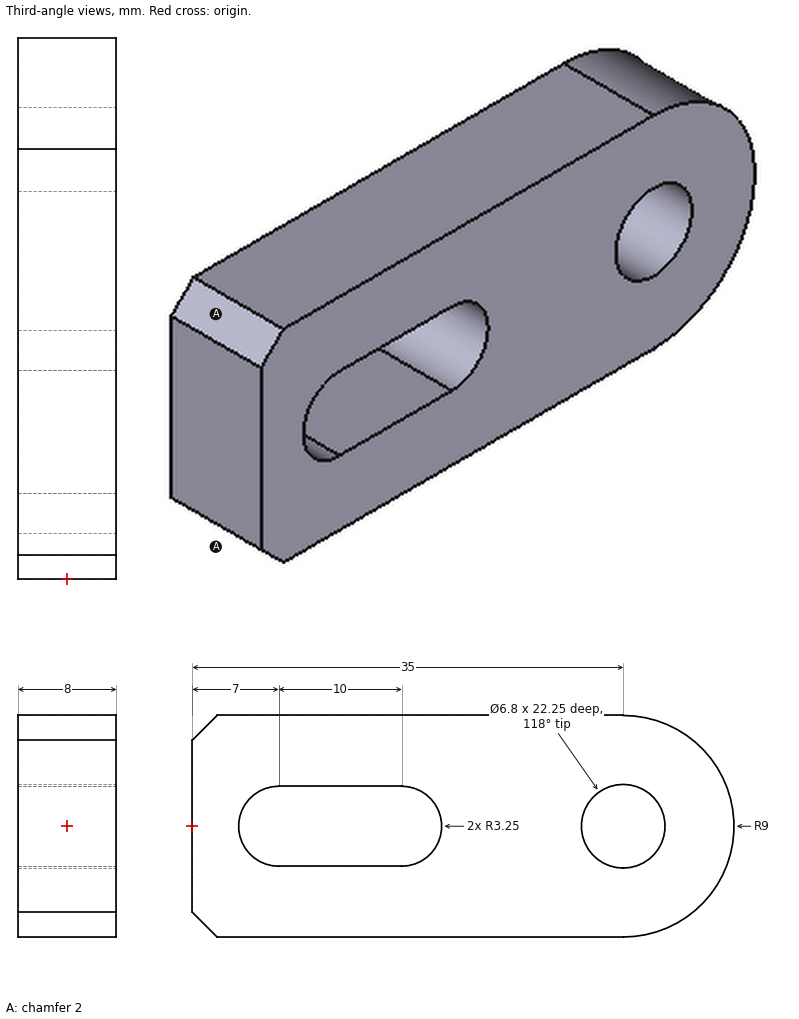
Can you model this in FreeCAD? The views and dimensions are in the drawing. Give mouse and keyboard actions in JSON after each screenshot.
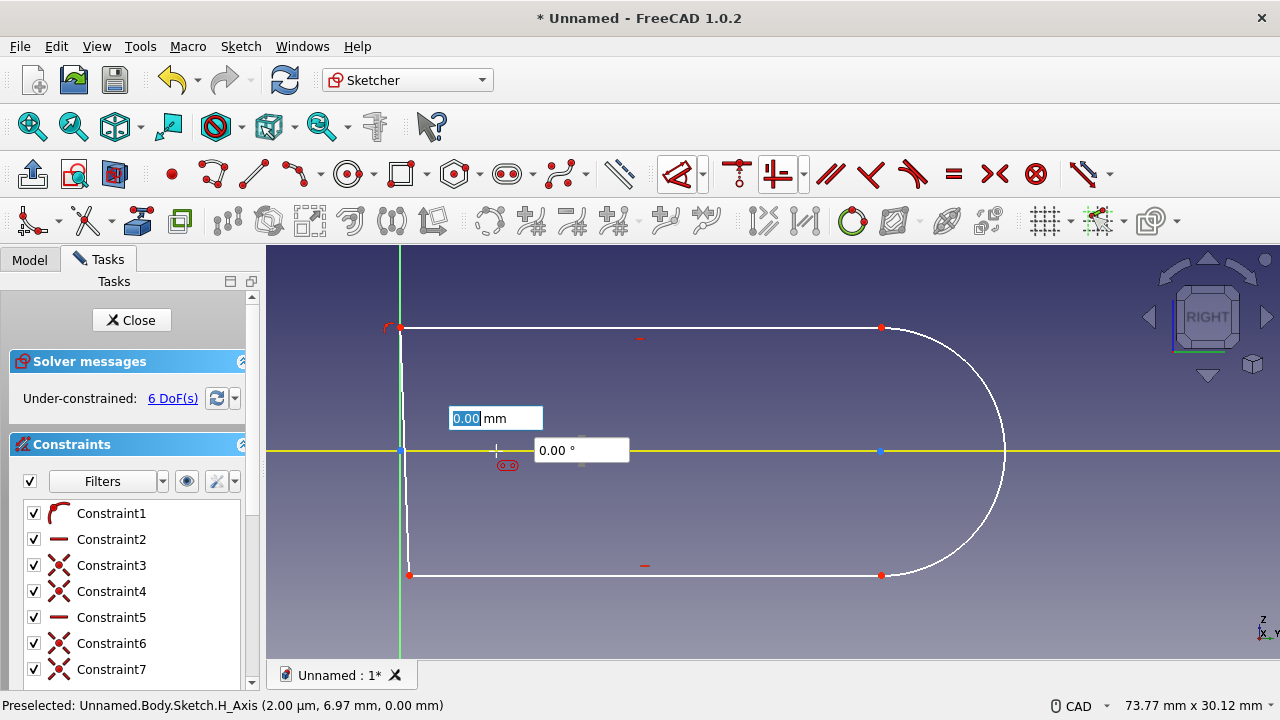
{"action": "left_click", "coordinate": [634, 442]}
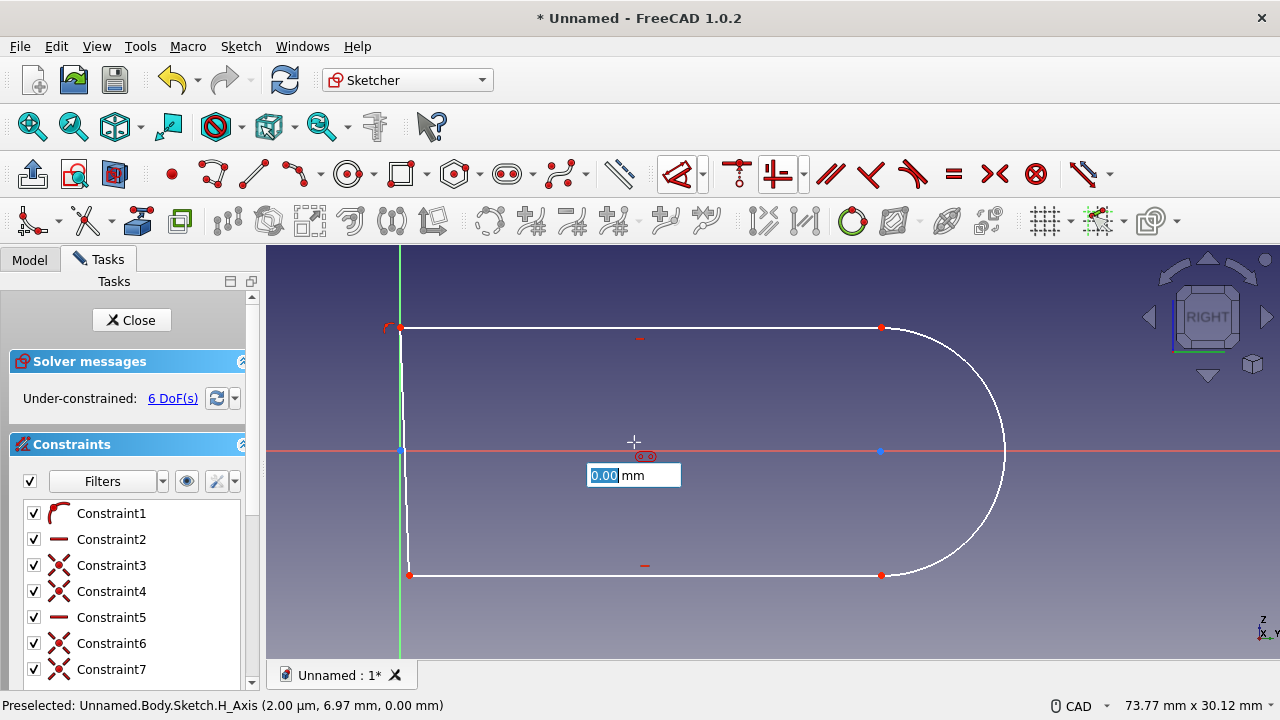
{"action": "left_click", "coordinate": [565, 496]}
{"action": "key", "text": "Escape"}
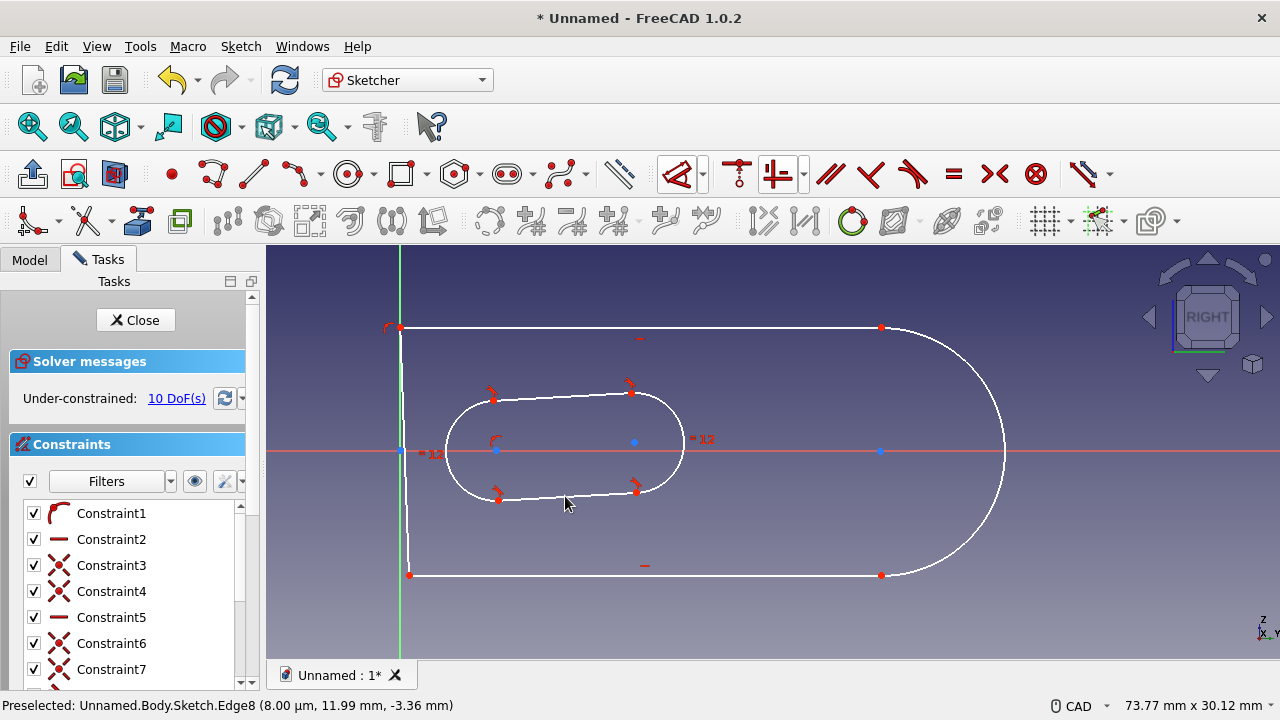
{"action": "left_click", "coordinate": [737, 328]}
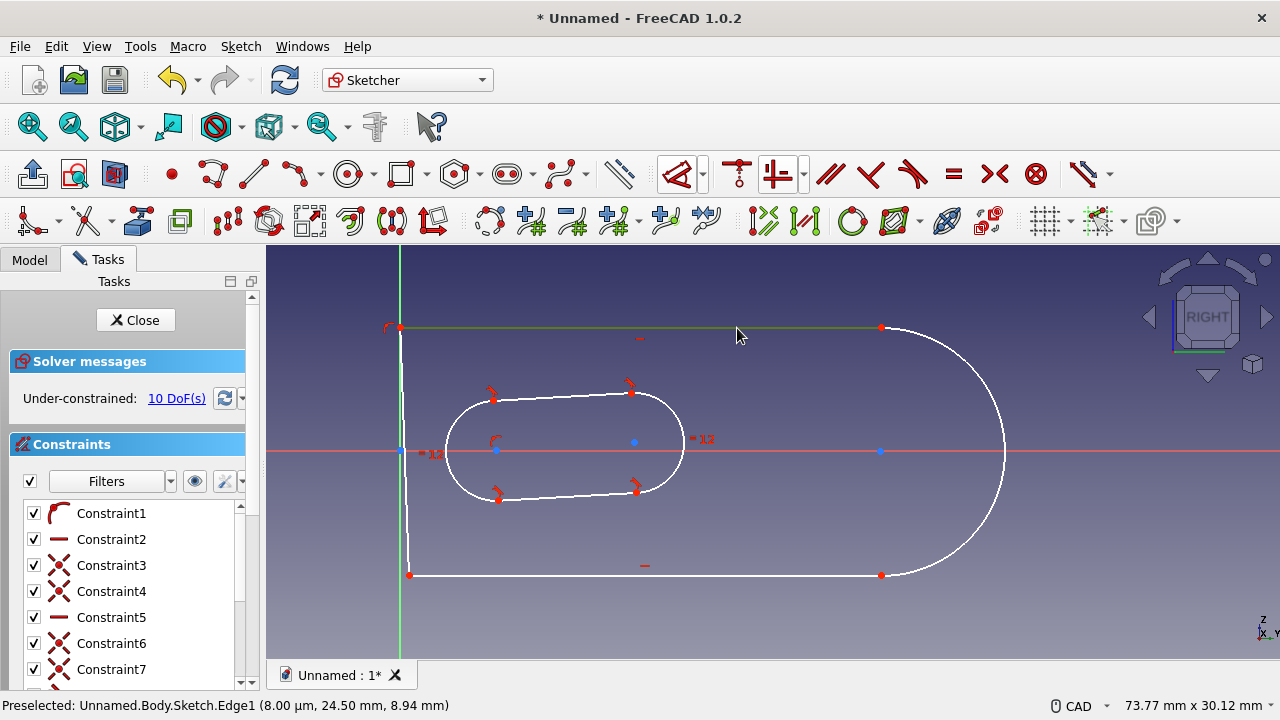
{"action": "left_click", "coordinate": [981, 525]}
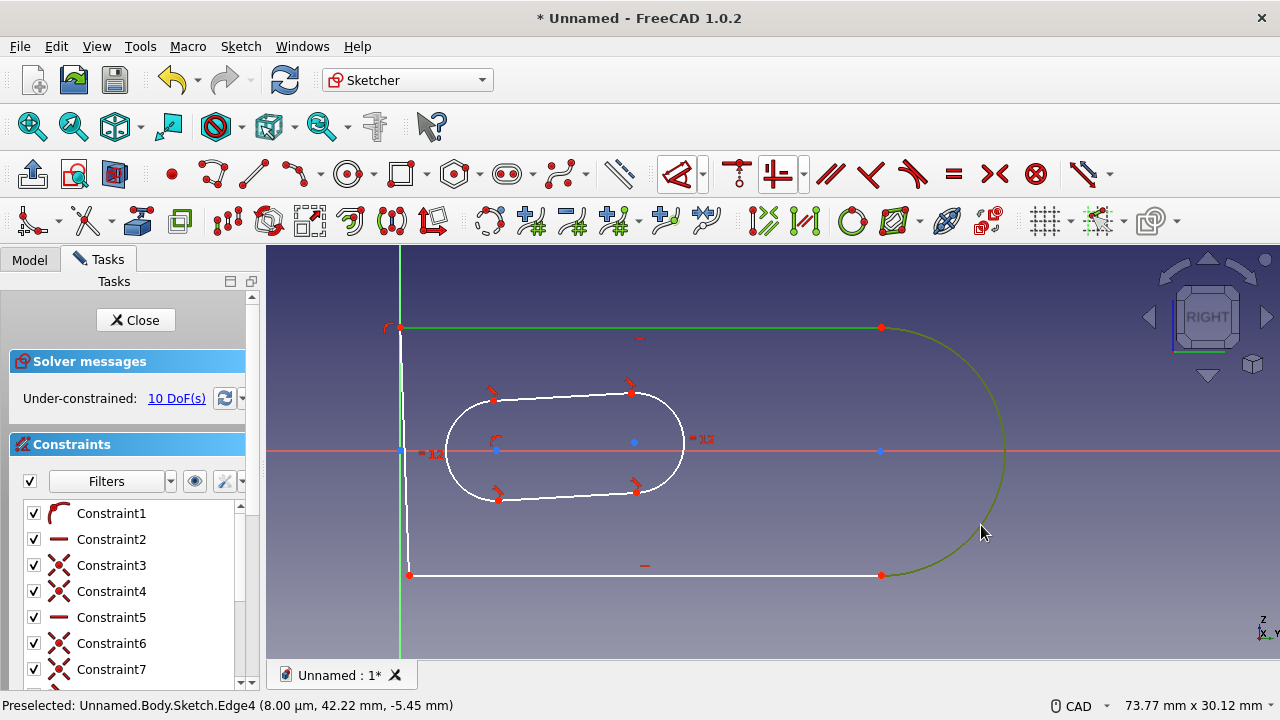
{"action": "key", "text": "t"}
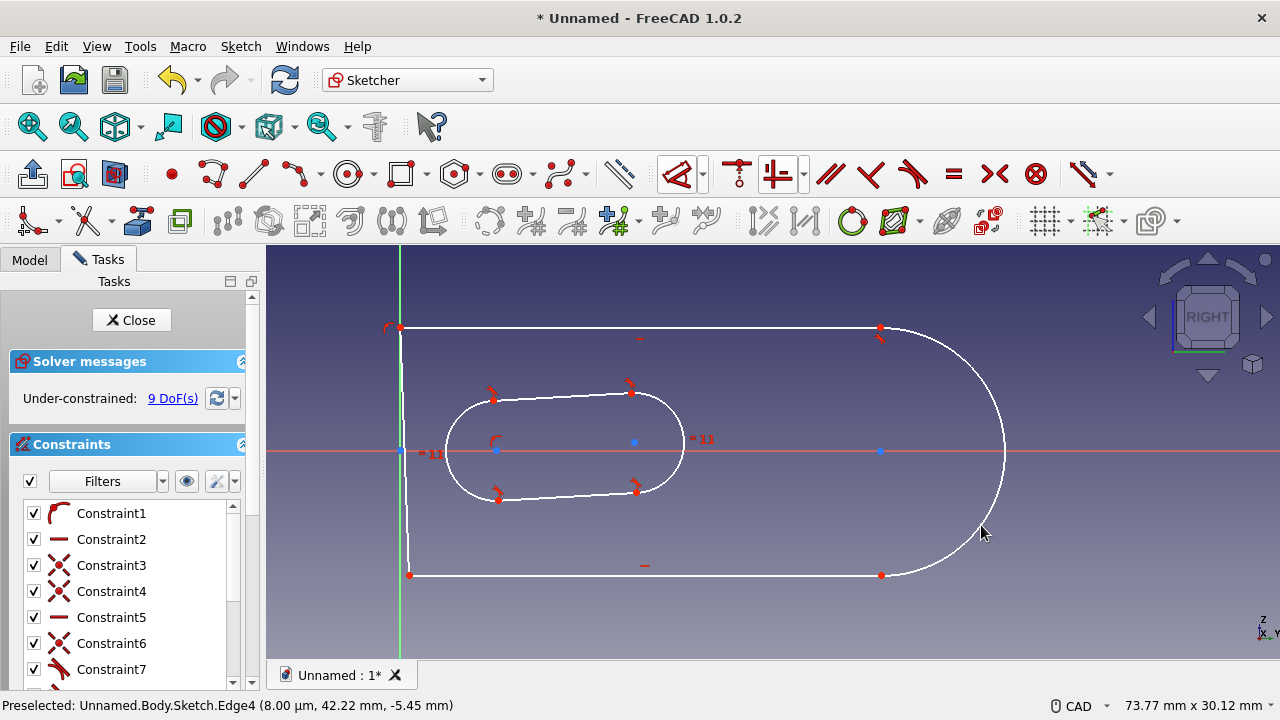
{"action": "left_click", "coordinate": [551, 576]}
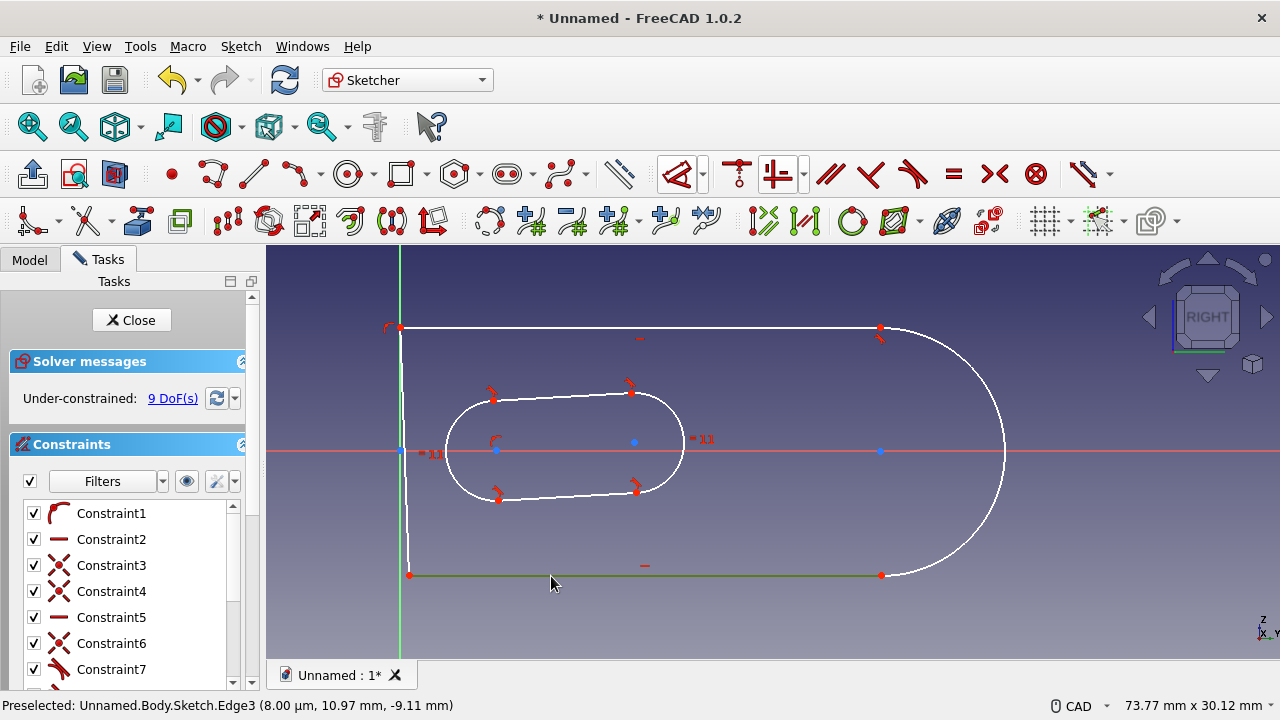
{"action": "left_click", "coordinate": [981, 525]}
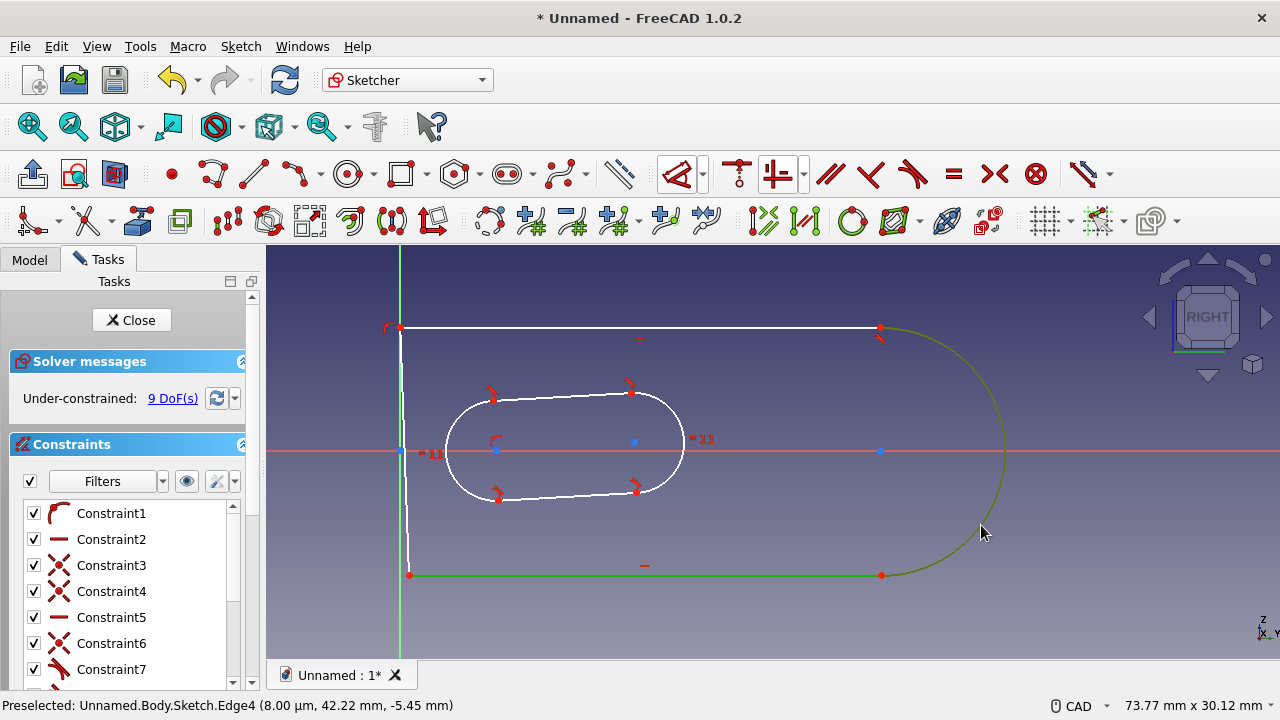
{"action": "key", "text": "t"}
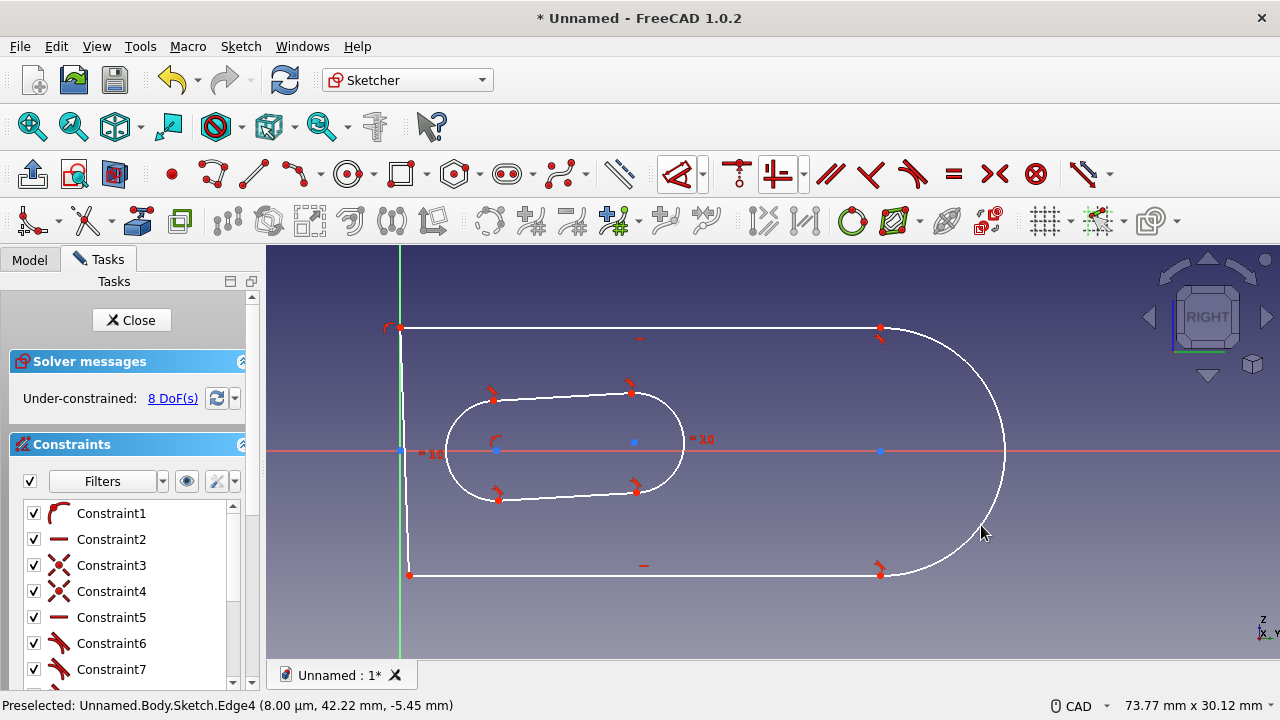
{"action": "left_click", "coordinate": [403, 402]}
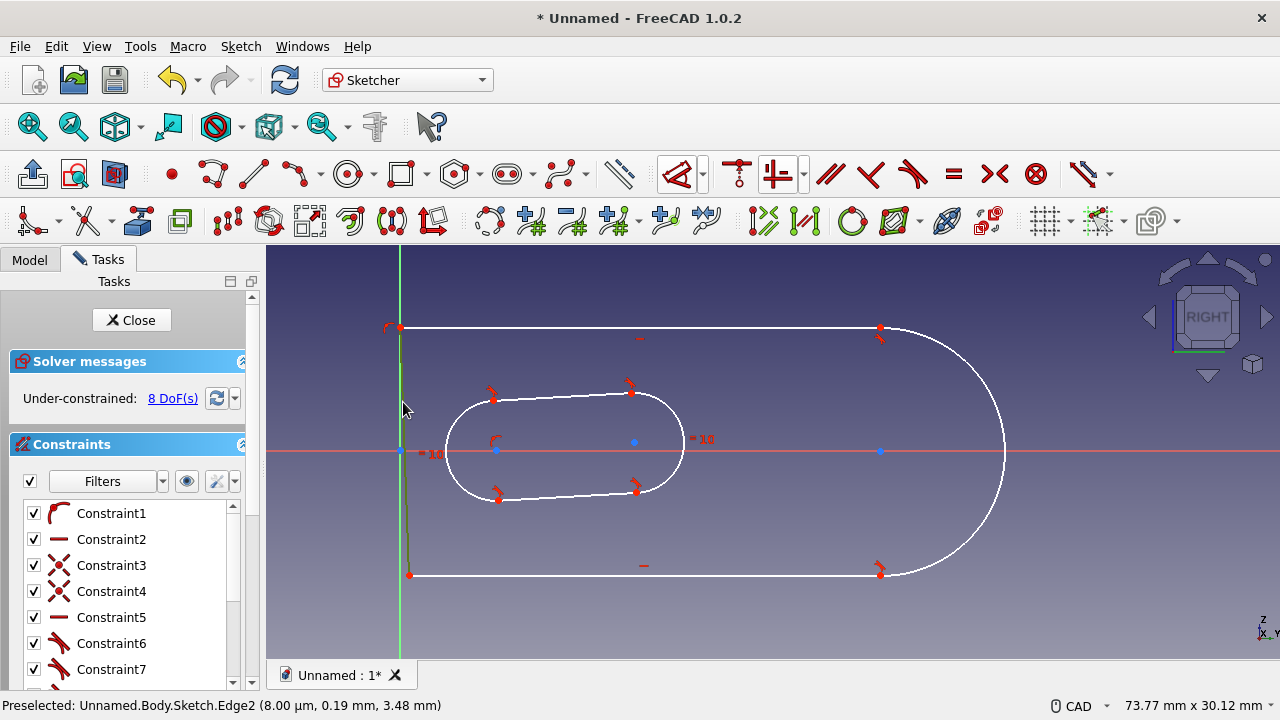
{"action": "key", "text": "v"}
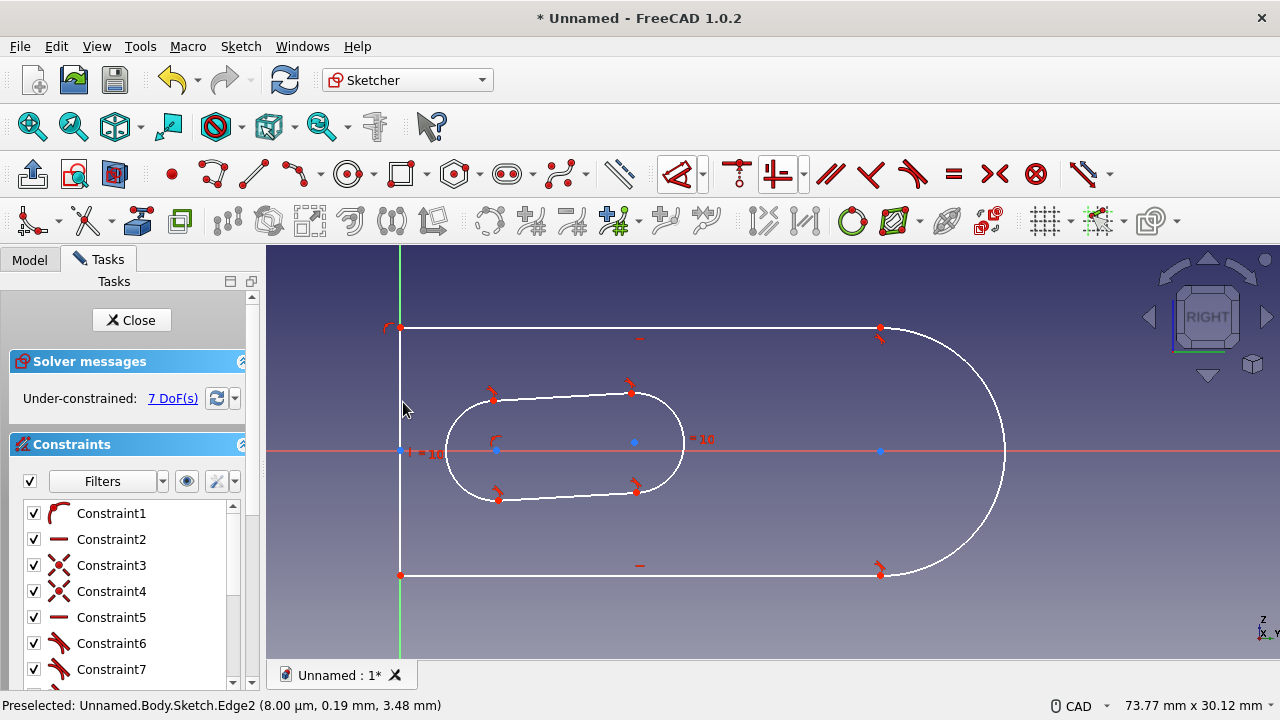
{"action": "left_click", "coordinate": [535, 399]}